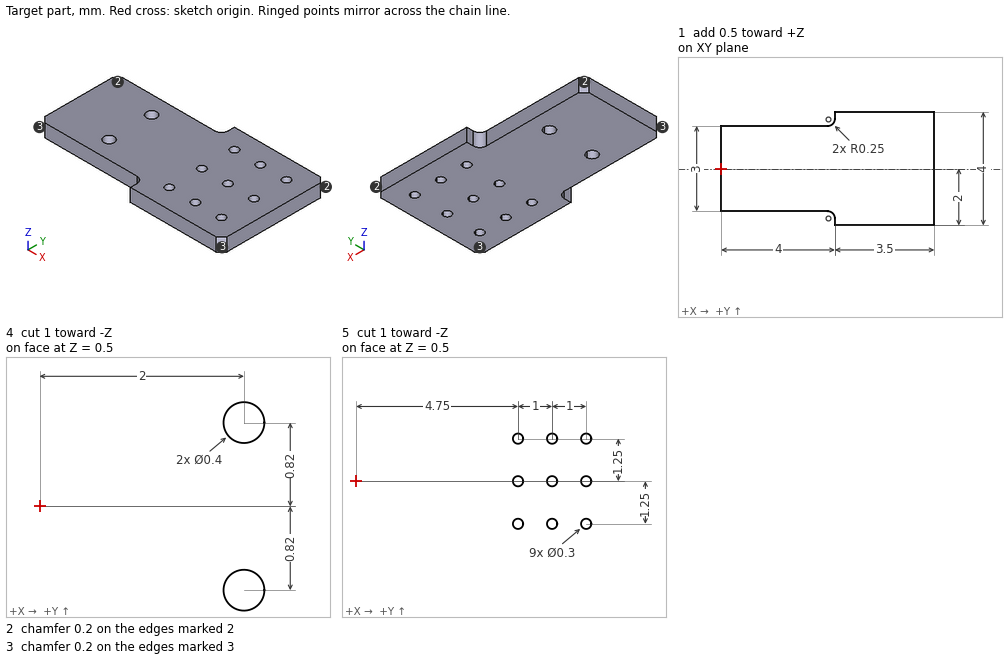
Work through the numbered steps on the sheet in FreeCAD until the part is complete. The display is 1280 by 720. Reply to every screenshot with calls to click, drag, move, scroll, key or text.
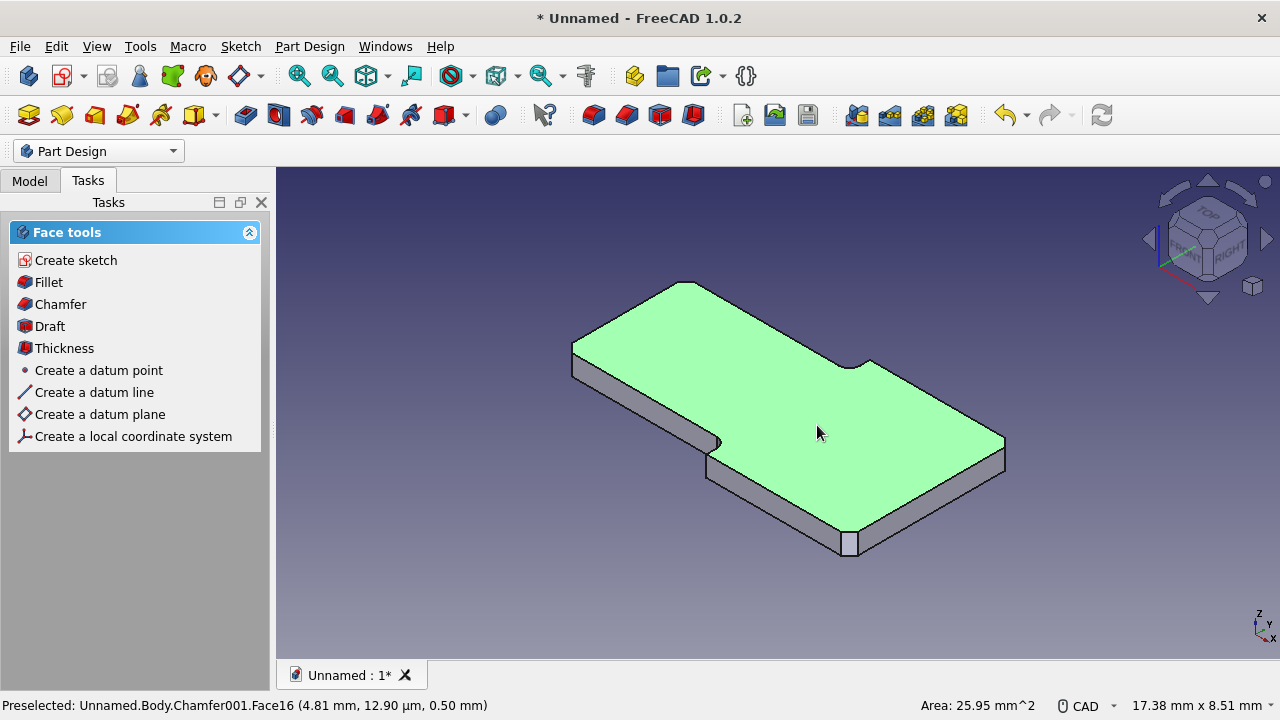
click(62, 76)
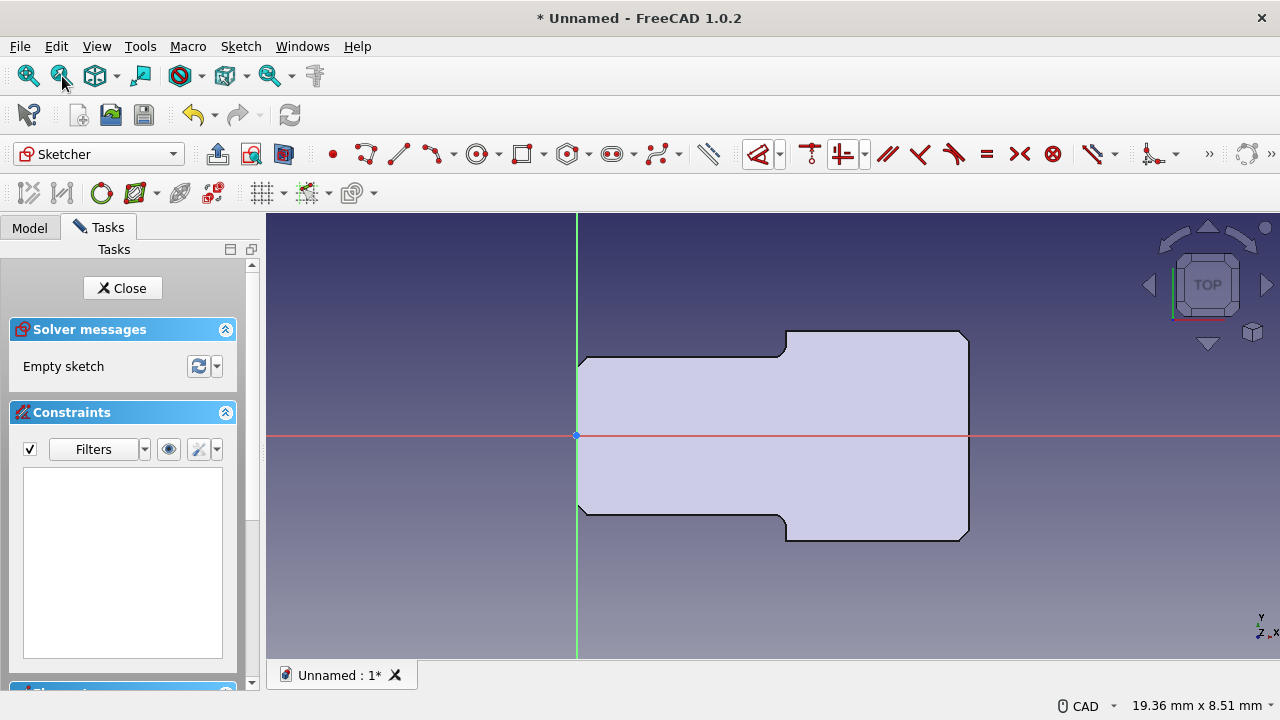
scroll(593, 436, up, 5)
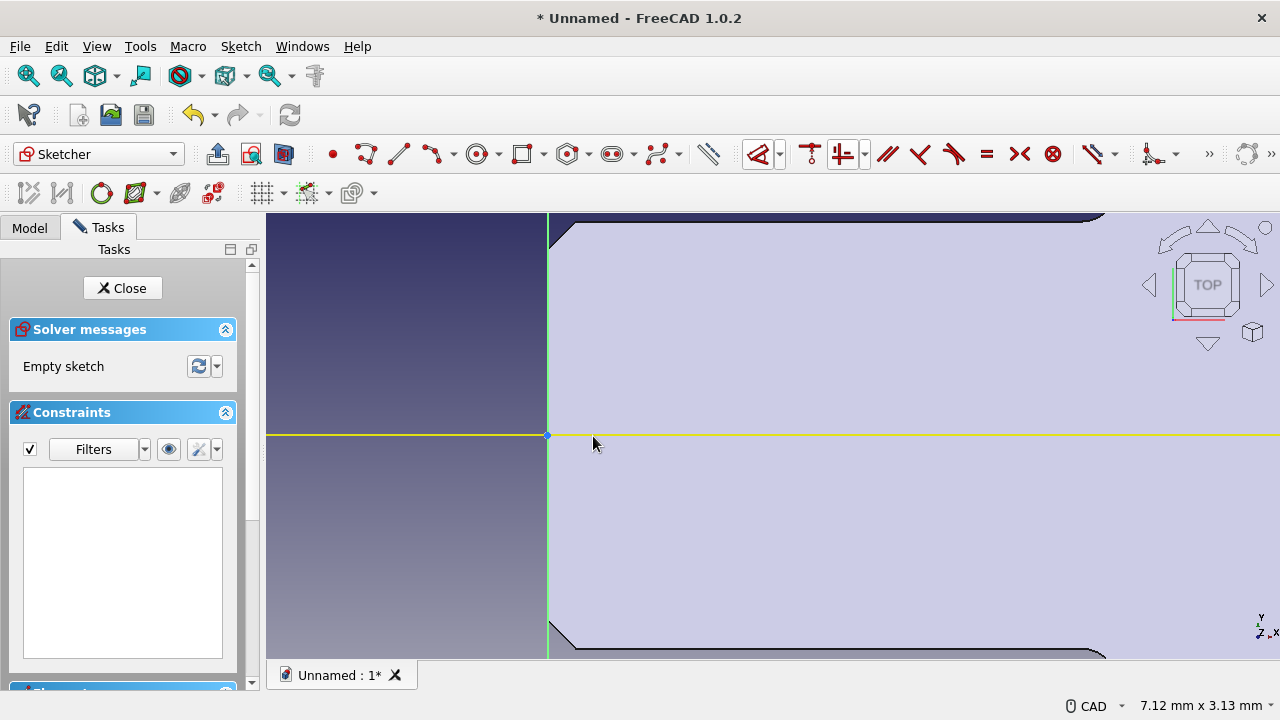
key(g)
key(c)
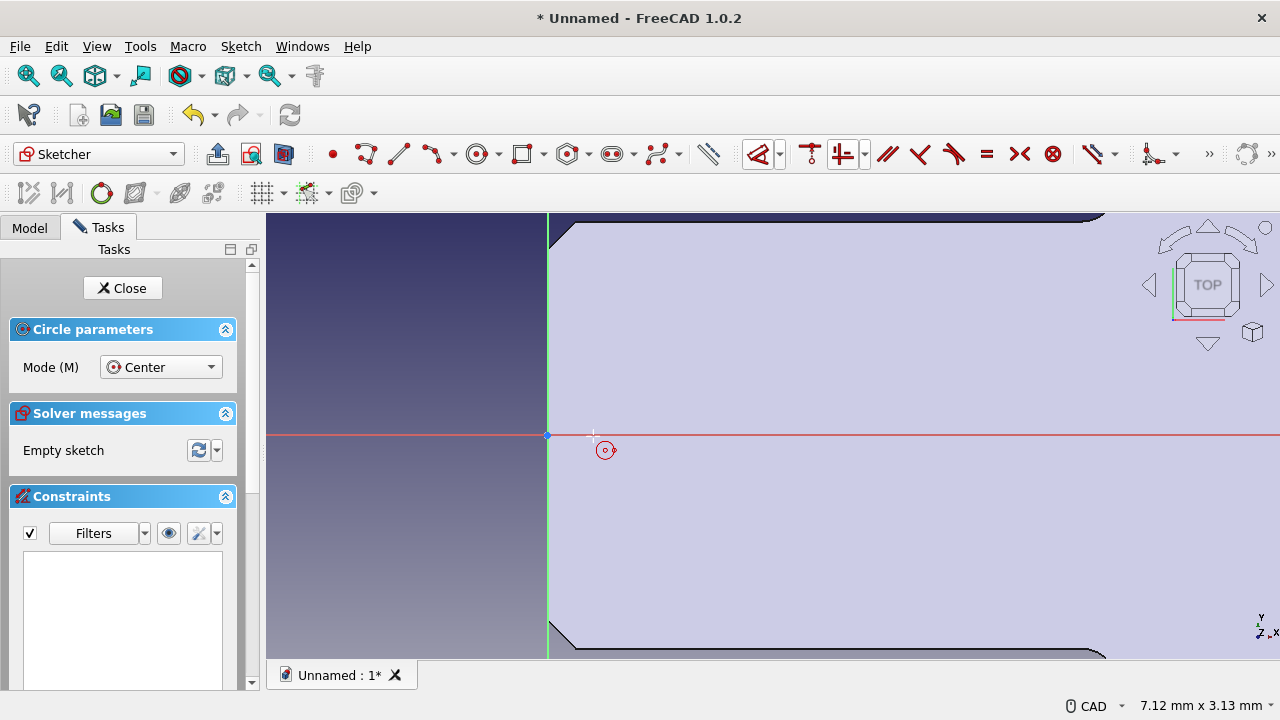
click(833, 318)
click(853, 298)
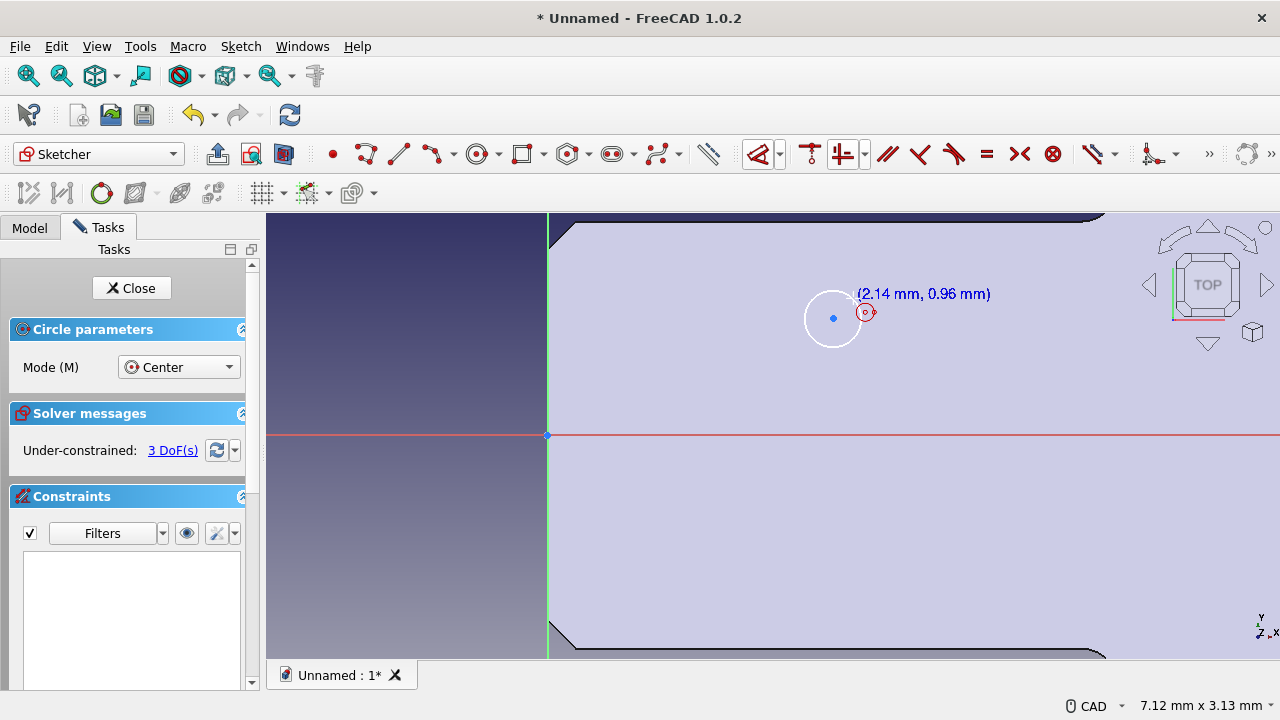
click(833, 552)
click(853, 532)
key(Escape)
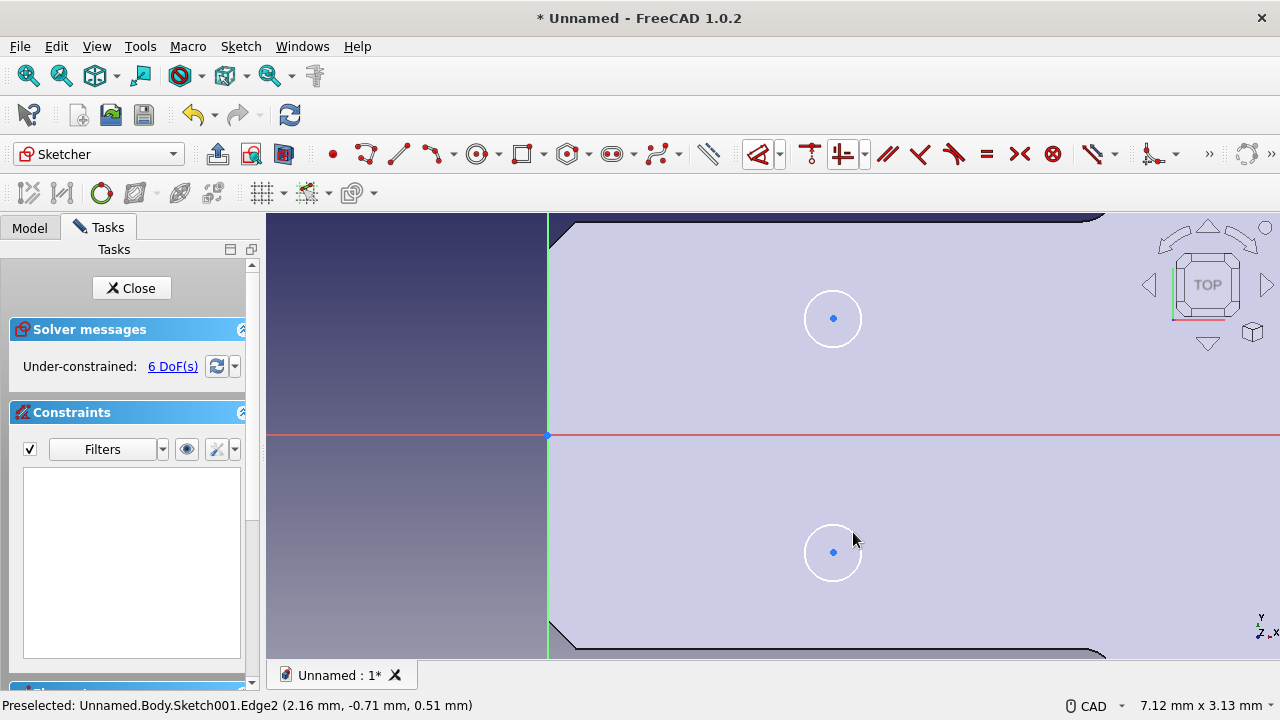
click(853, 299)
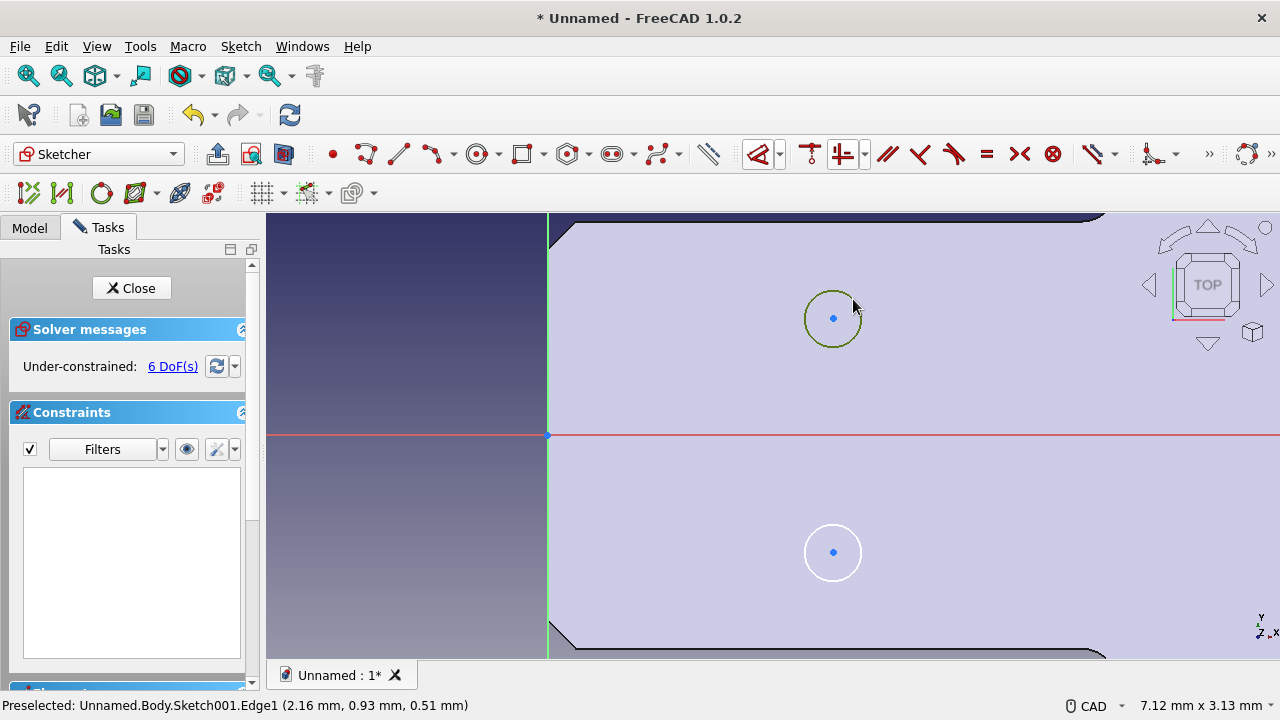
click(853, 533)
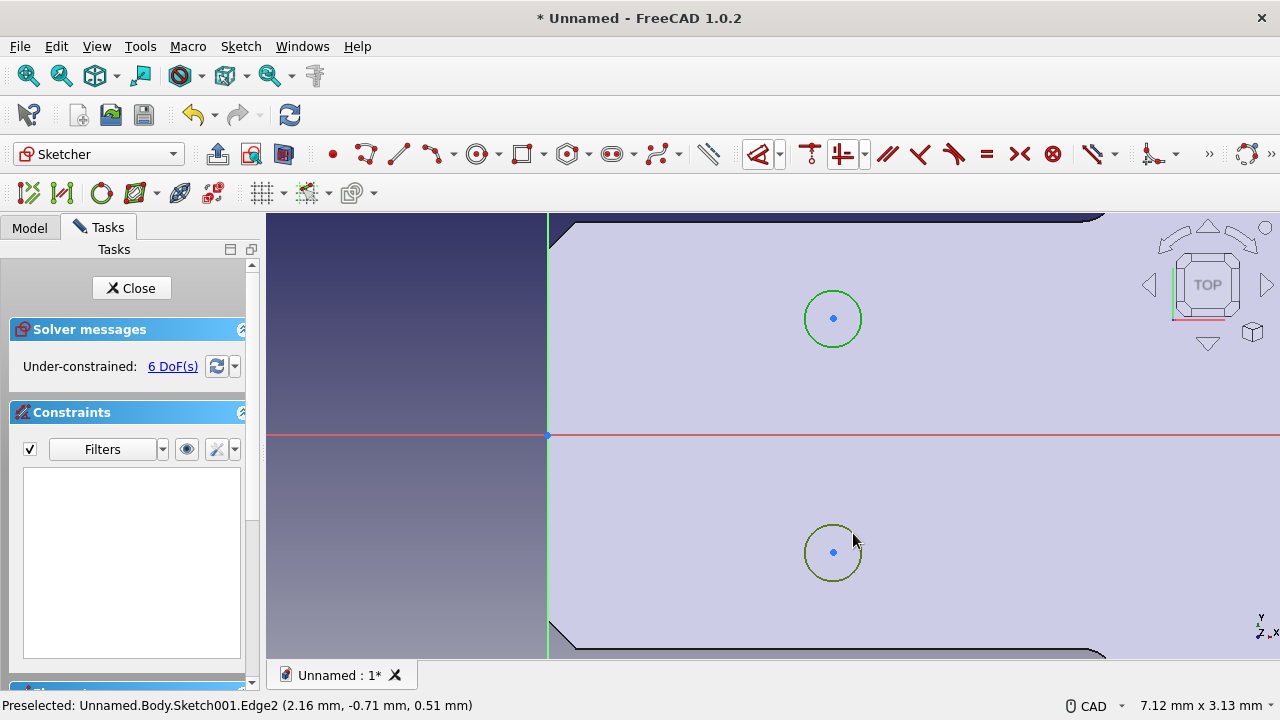
key(e)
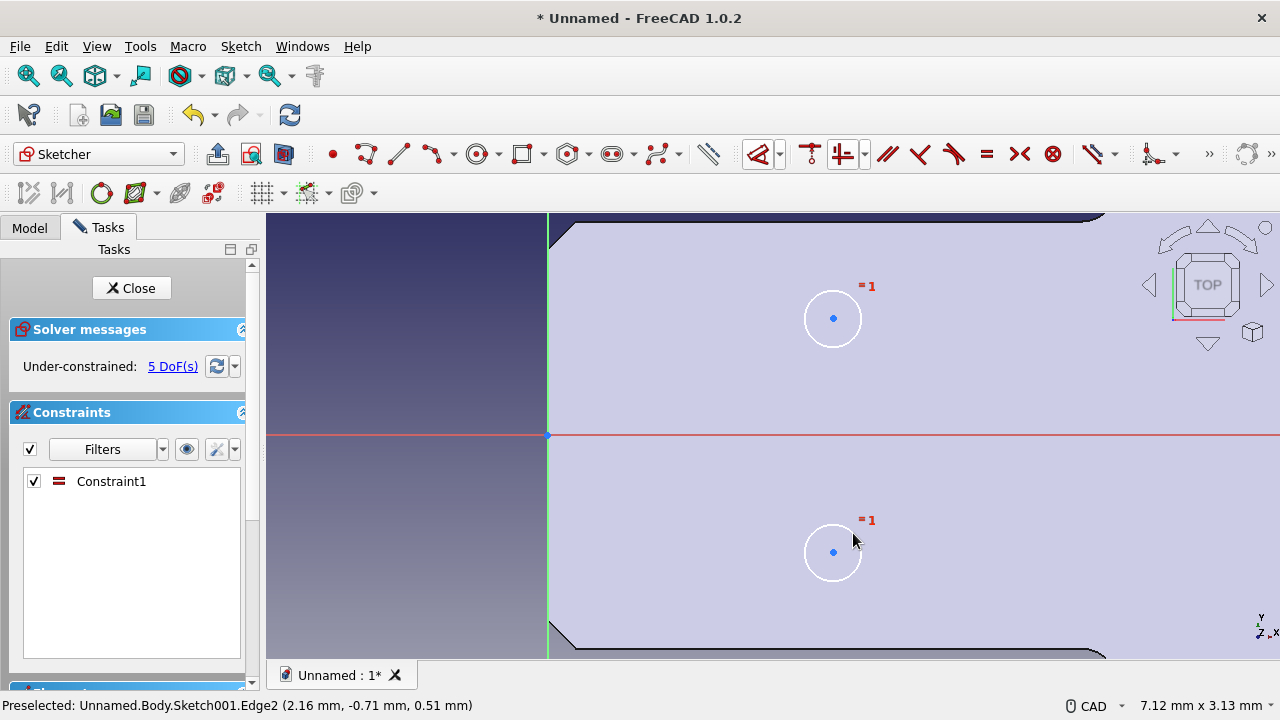
click(833, 319)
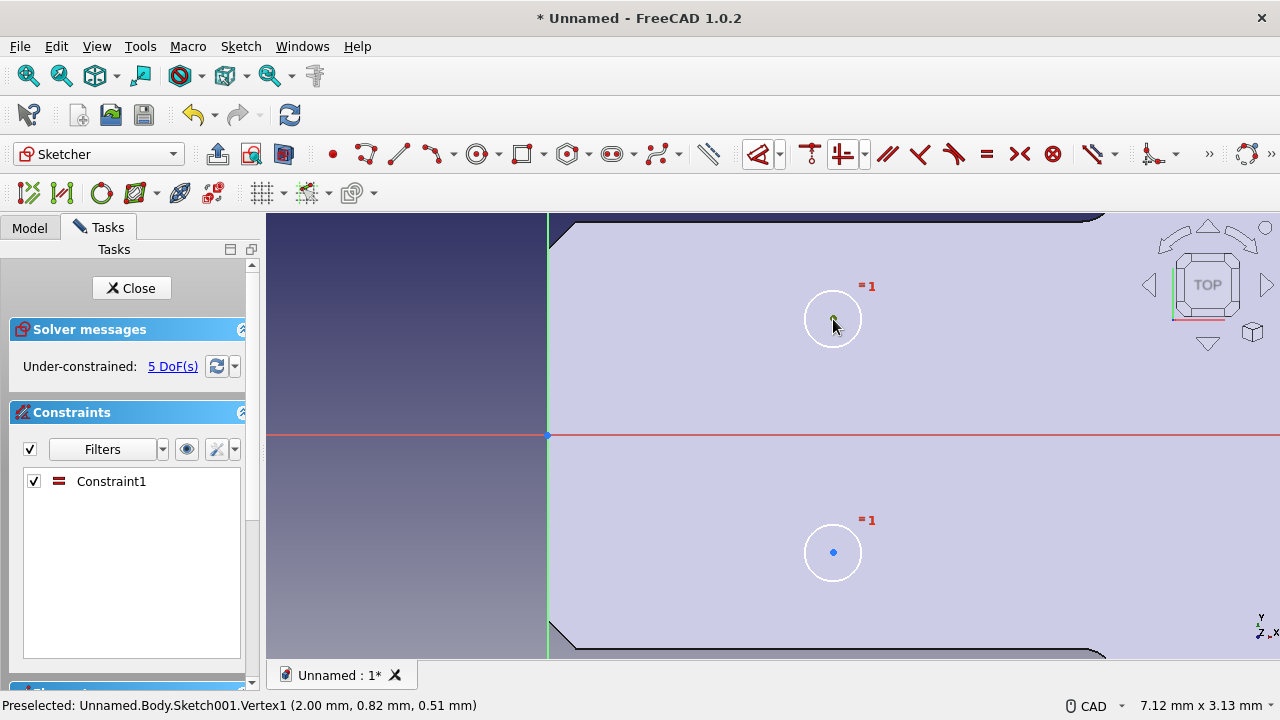
click(833, 553)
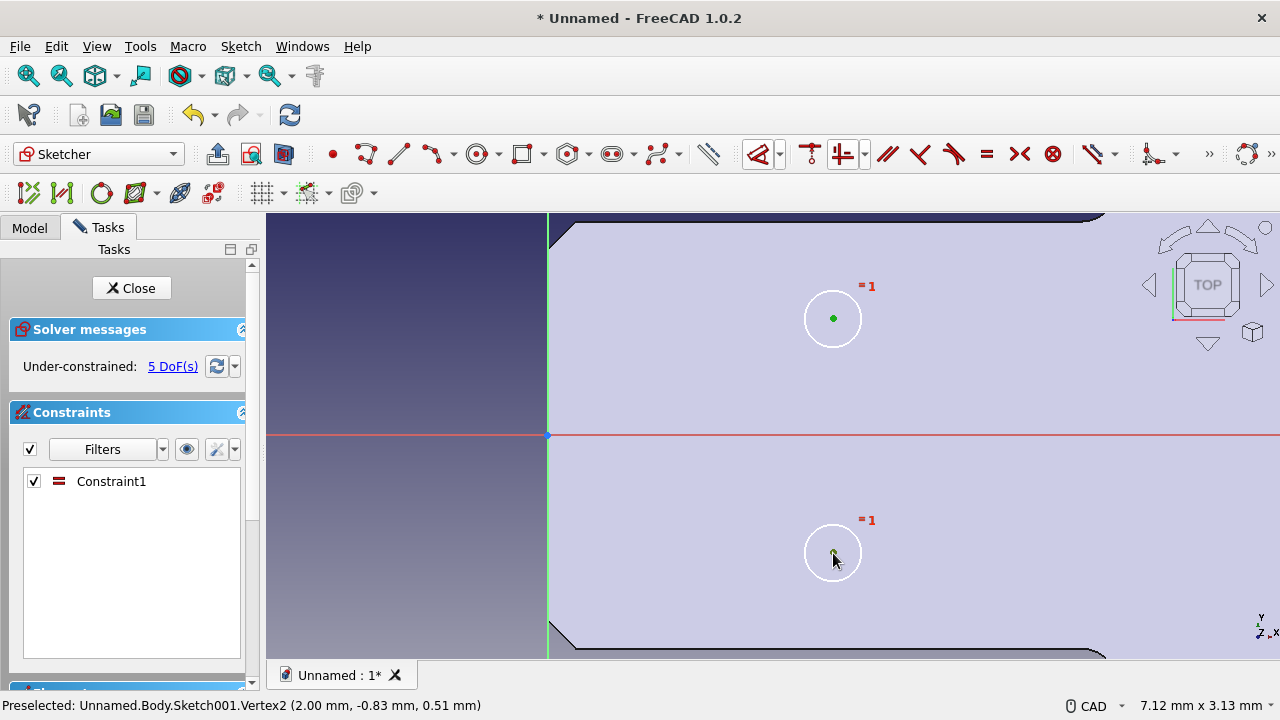
key(v)